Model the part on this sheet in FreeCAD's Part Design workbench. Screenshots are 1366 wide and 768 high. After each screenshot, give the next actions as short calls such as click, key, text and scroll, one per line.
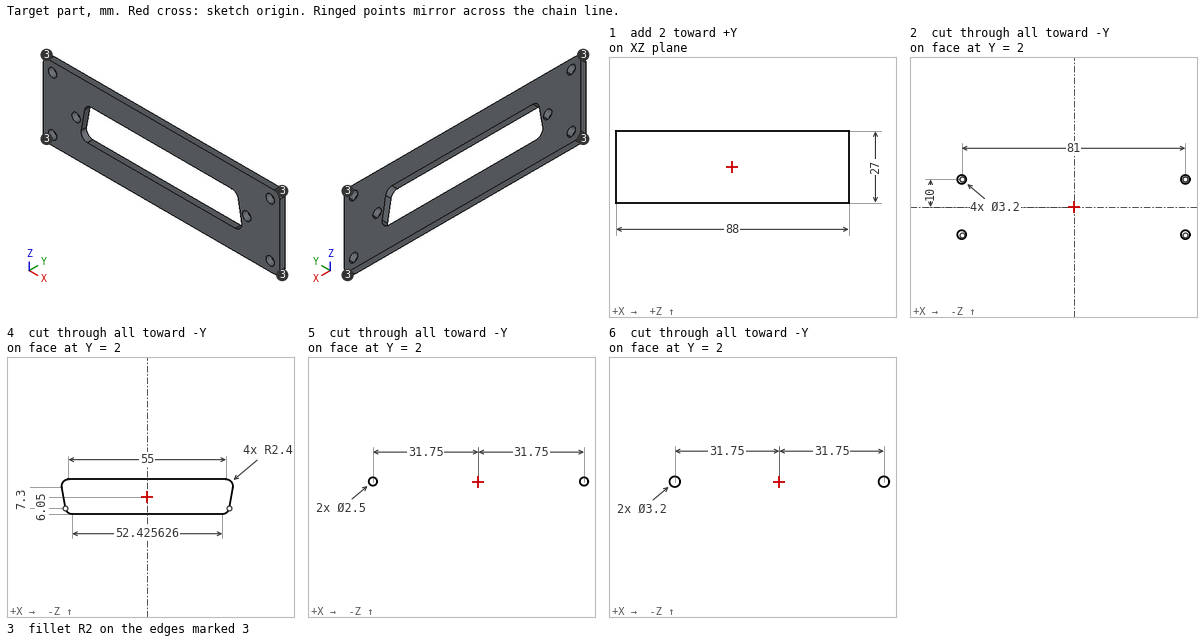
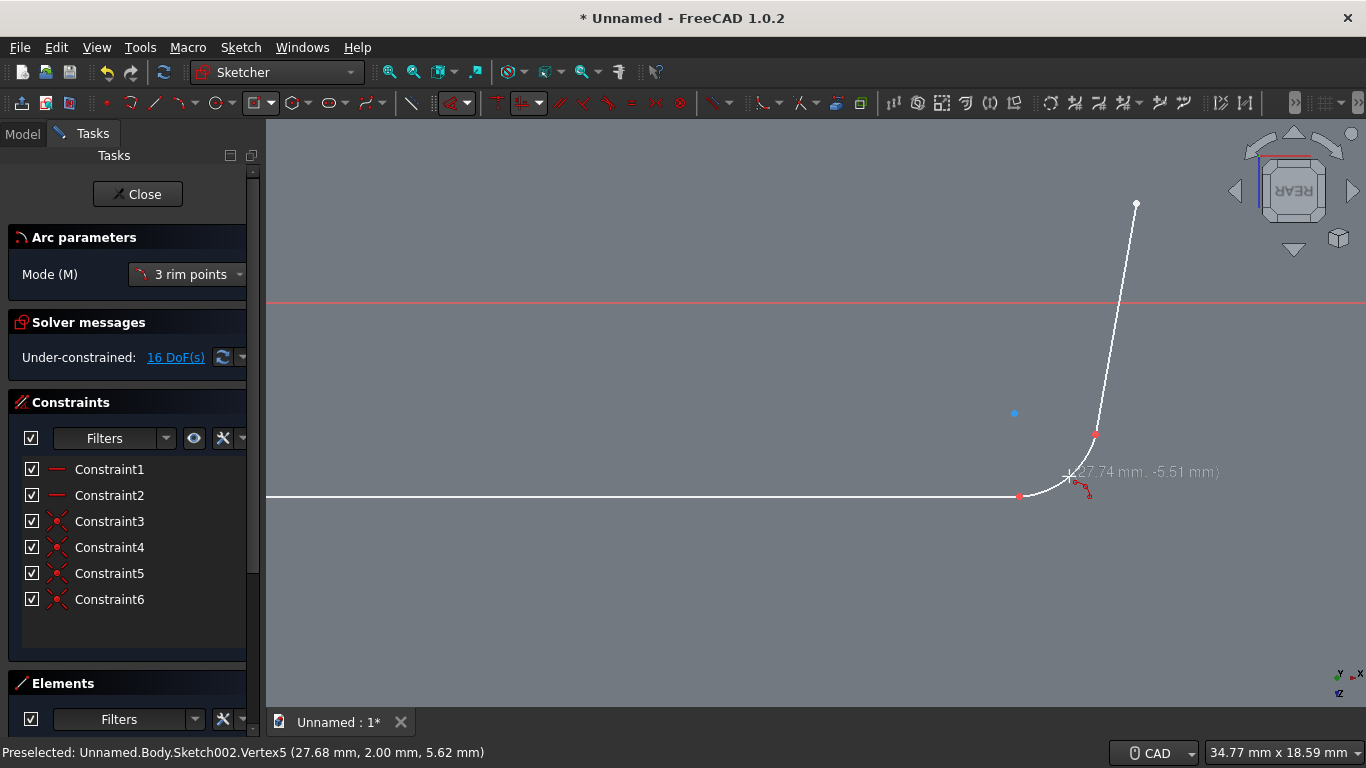
click(1137, 203)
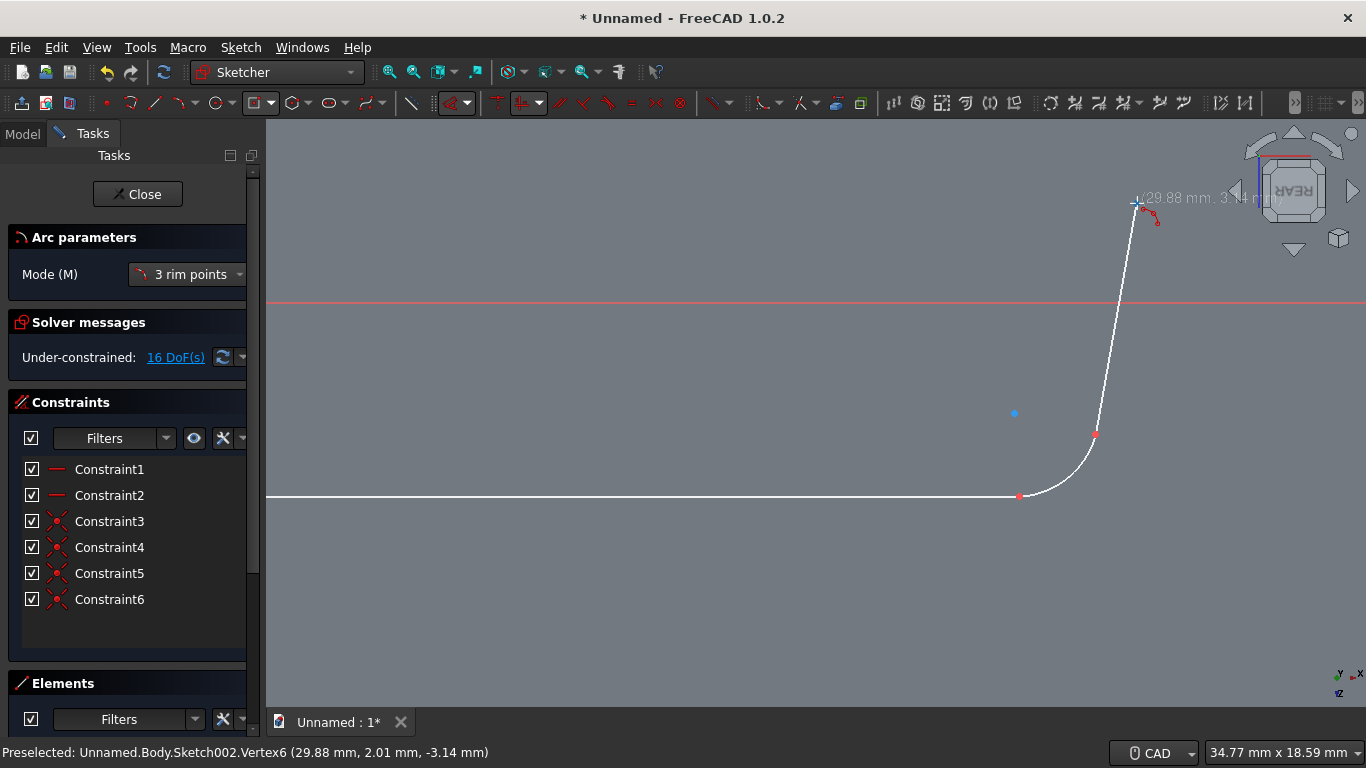
scroll(1071, 477, down, 5)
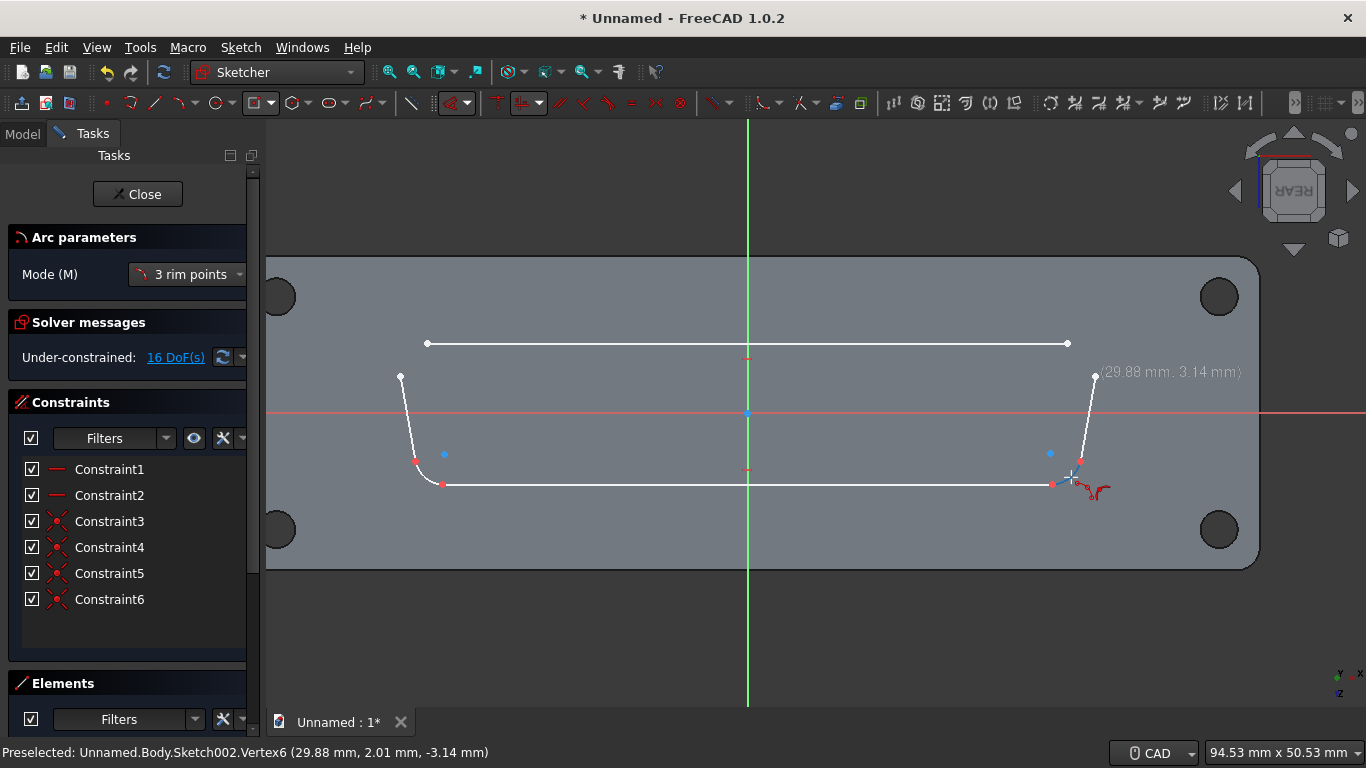
click(1068, 344)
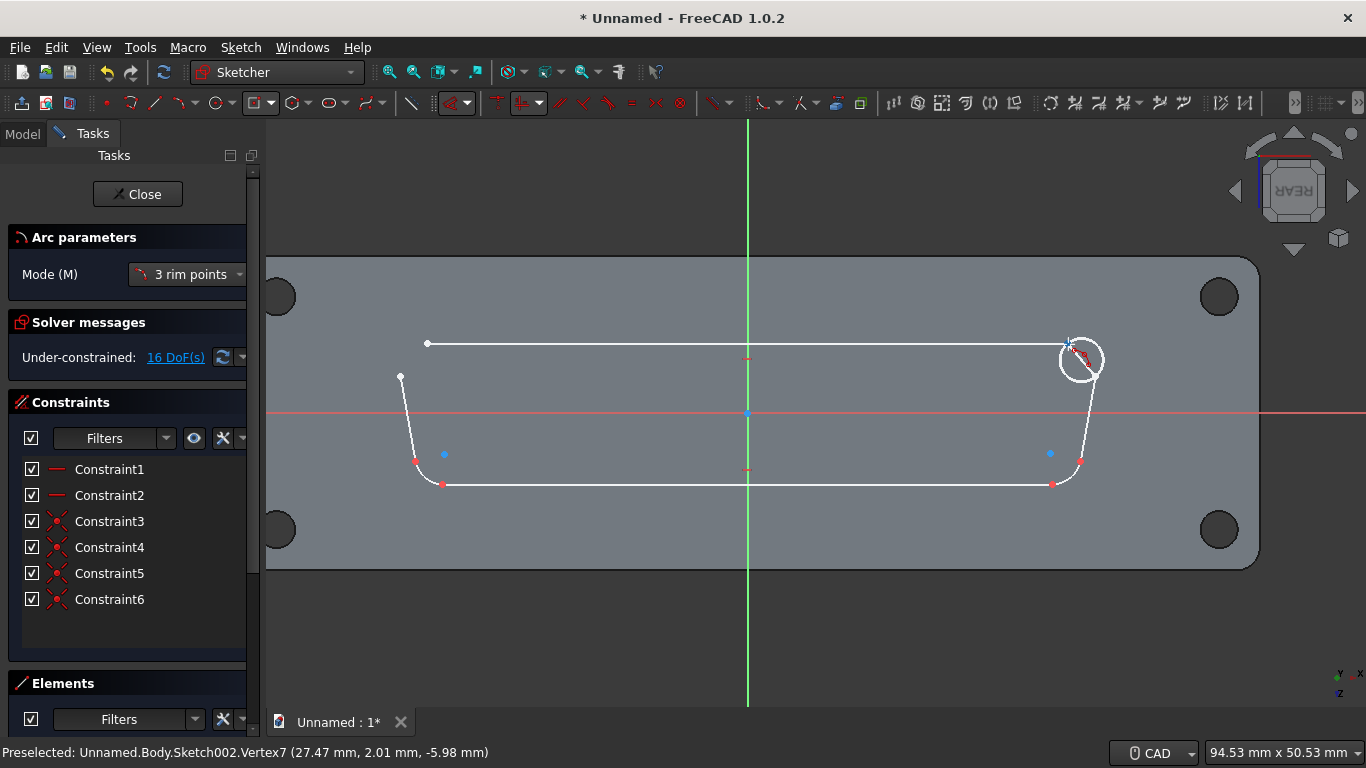
scroll(1089, 353, up, 3)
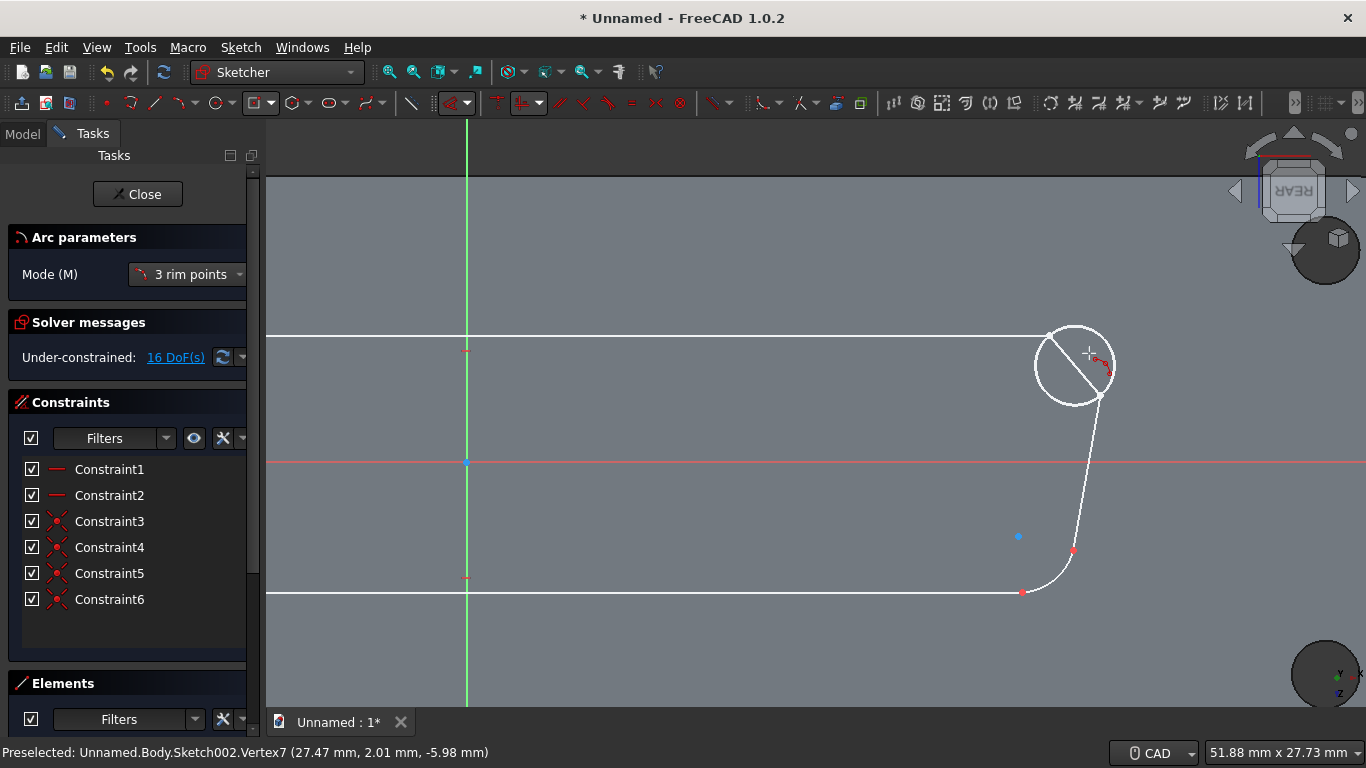
click(1089, 352)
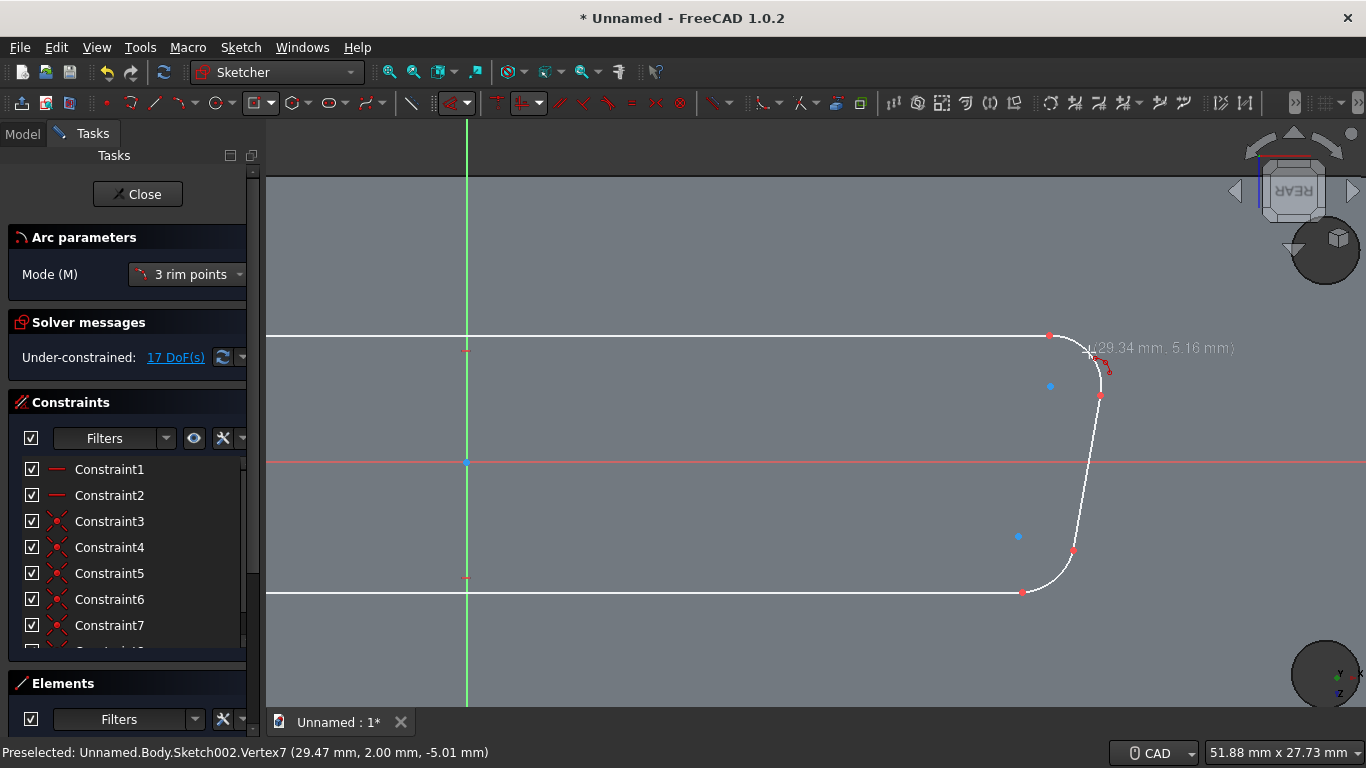
scroll(1089, 353, down, 3)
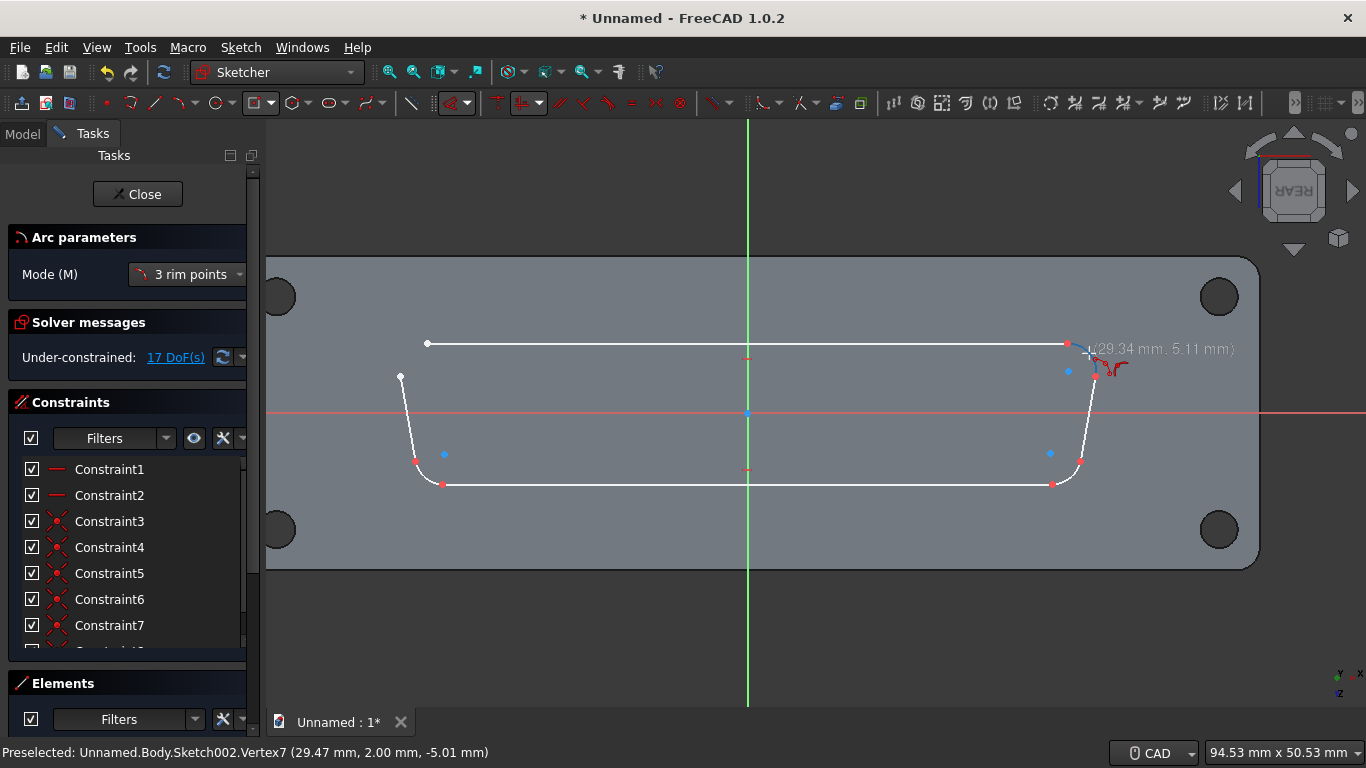
click(428, 344)
click(401, 377)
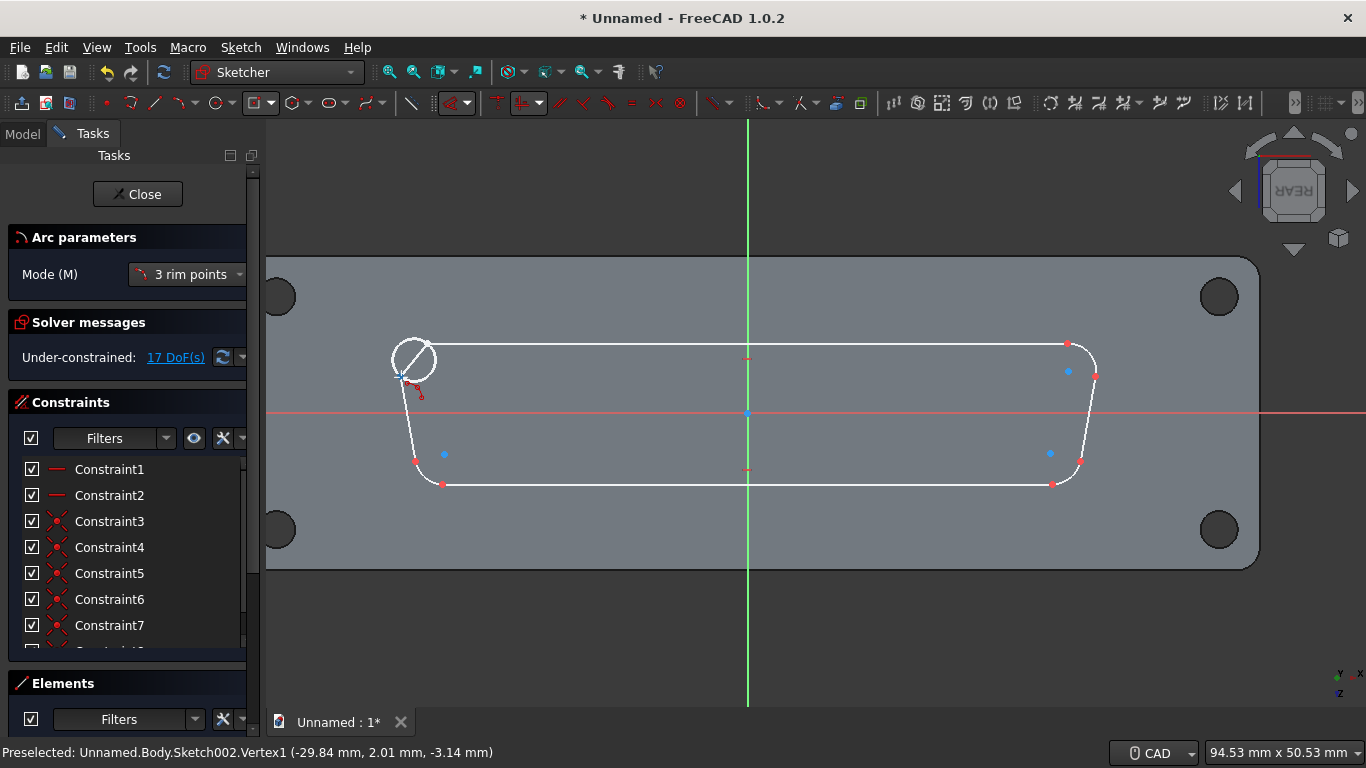
scroll(407, 353, up, 3)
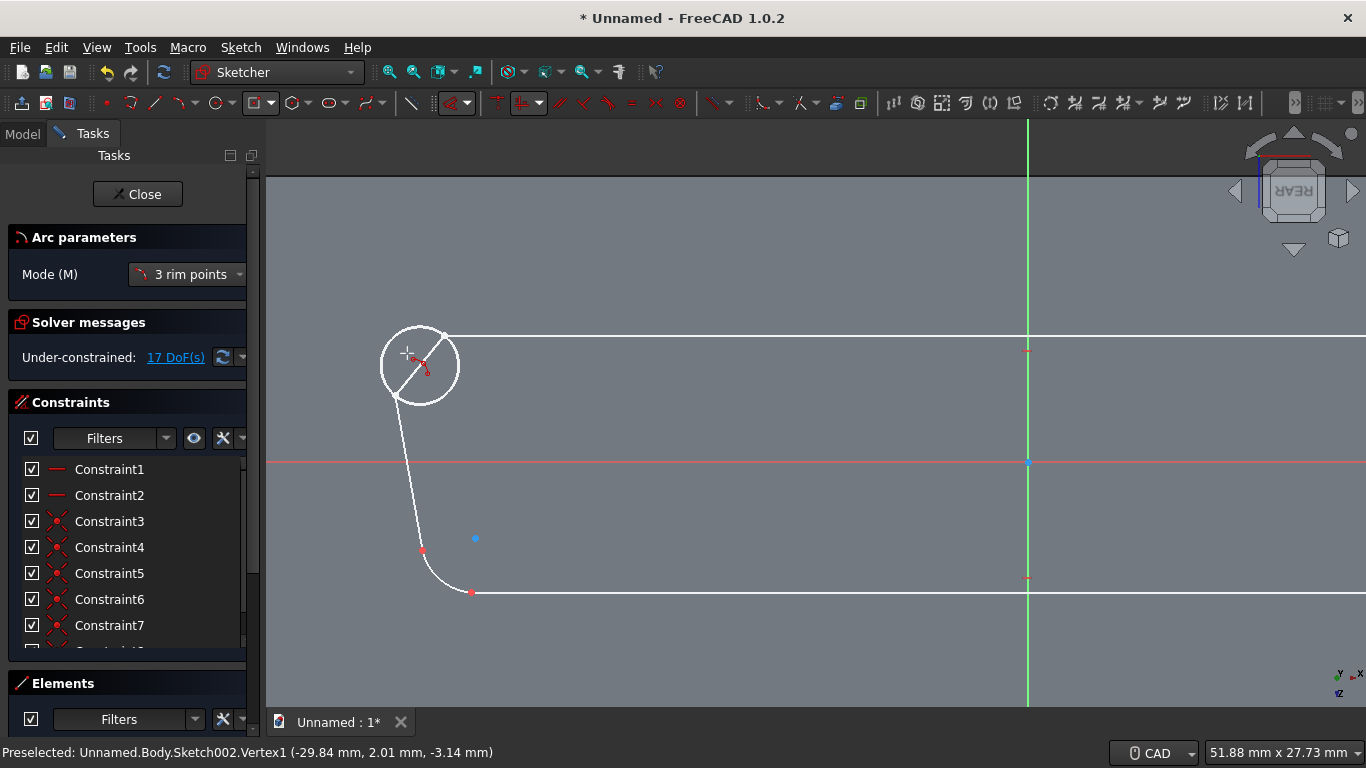
click(406, 352)
key(Escape)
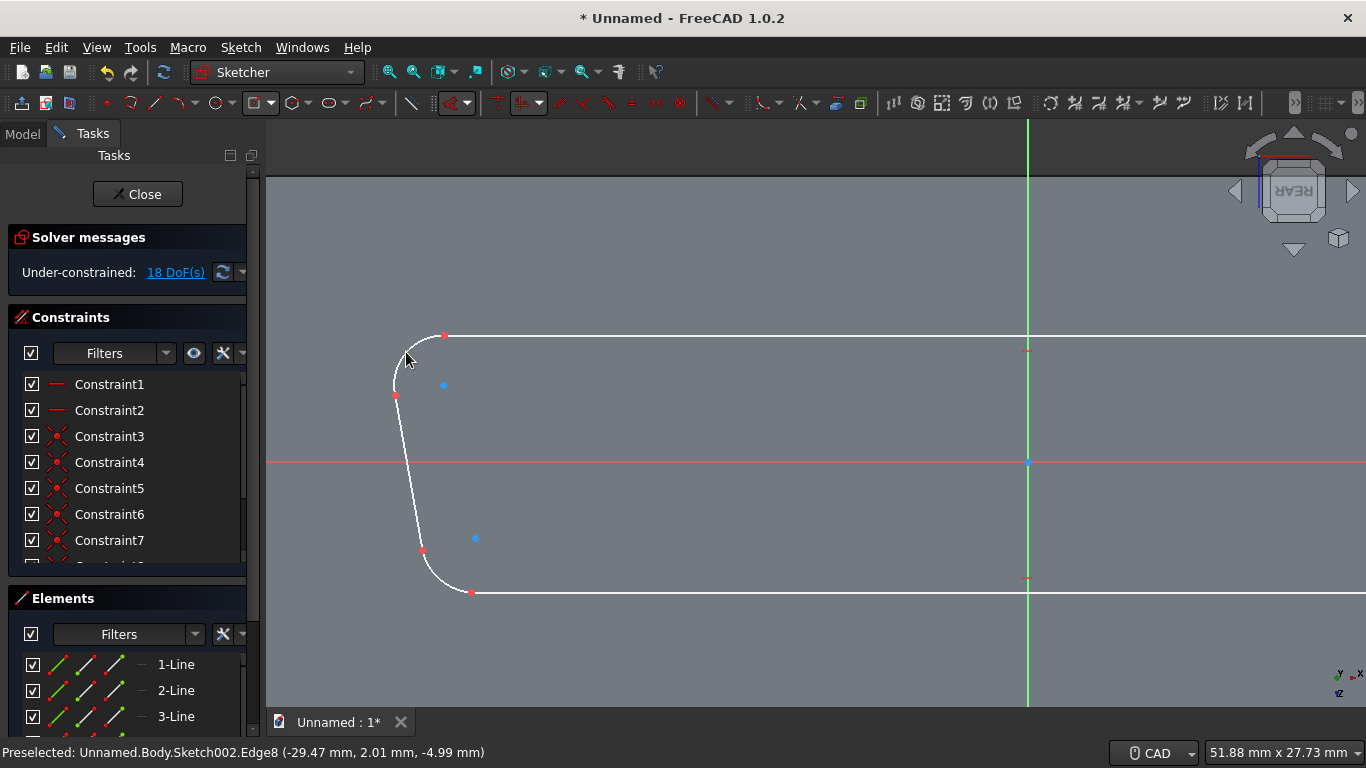
click(403, 442)